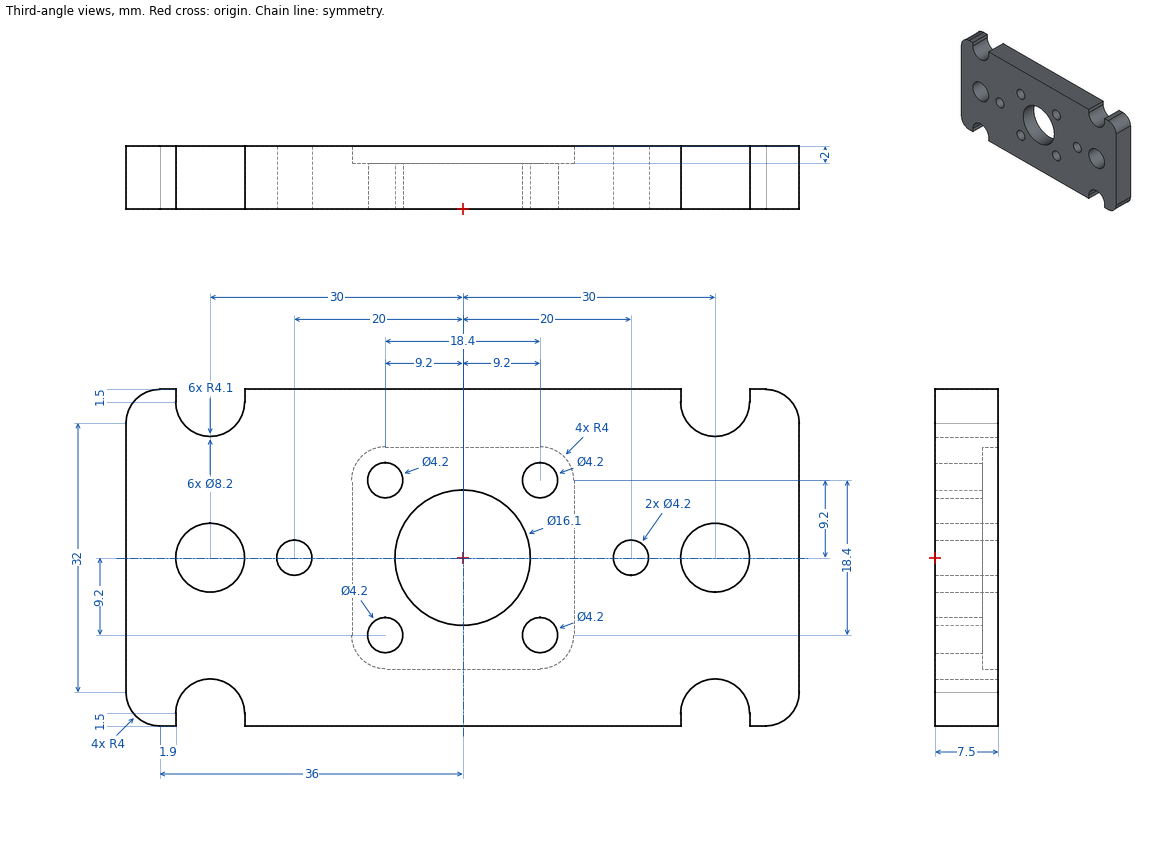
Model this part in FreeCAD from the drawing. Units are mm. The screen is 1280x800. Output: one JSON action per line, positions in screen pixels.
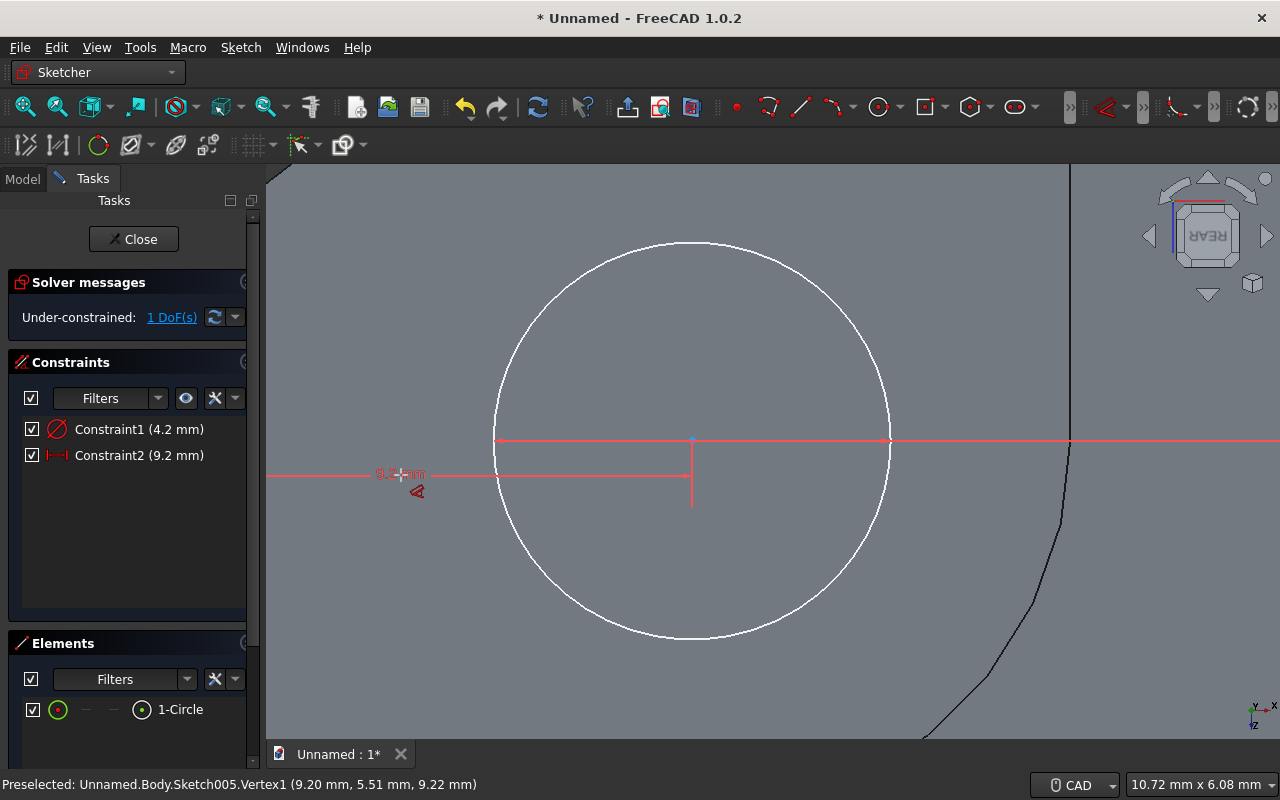
{"action": "left_click", "coordinate": [692, 441]}
{"action": "left_click", "coordinate": [726, 316]}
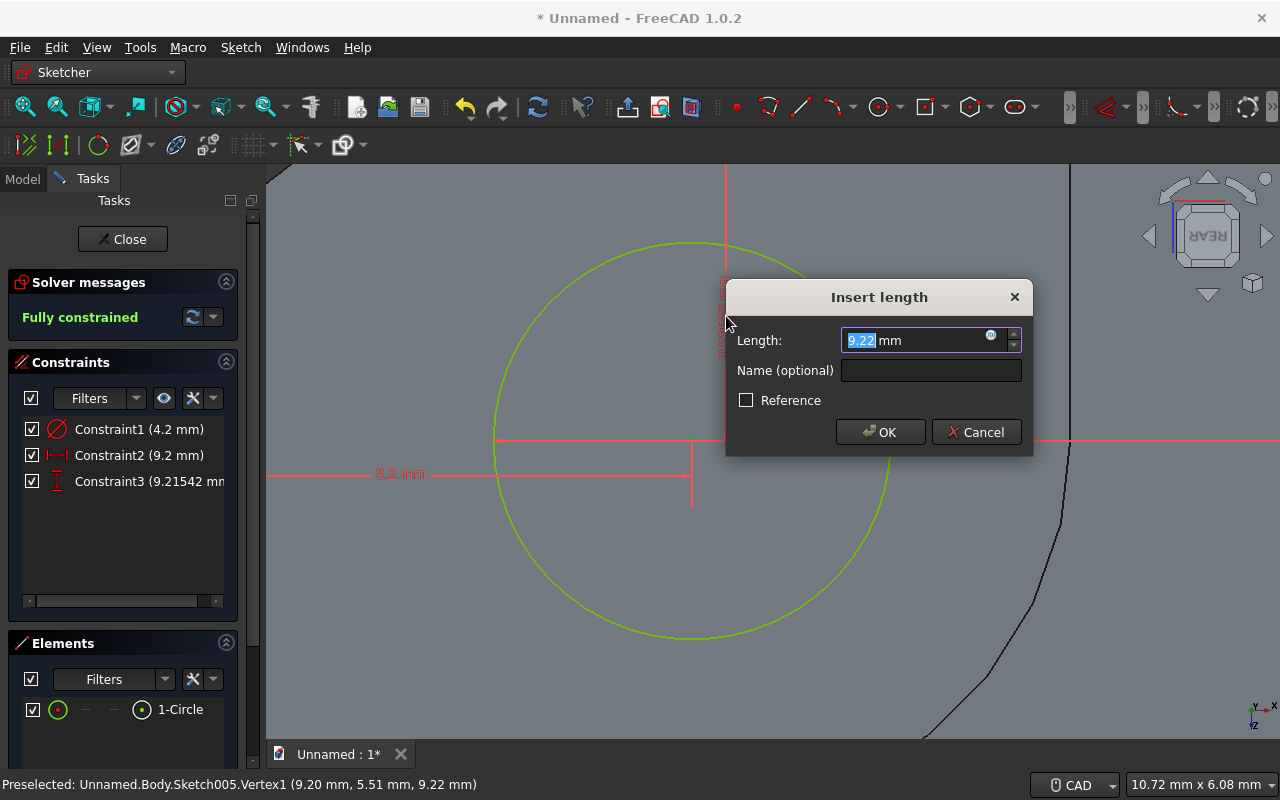
{"action": "type", "text": "9.2"}
{"action": "key", "text": "Return"}
{"action": "key", "text": "Escape"}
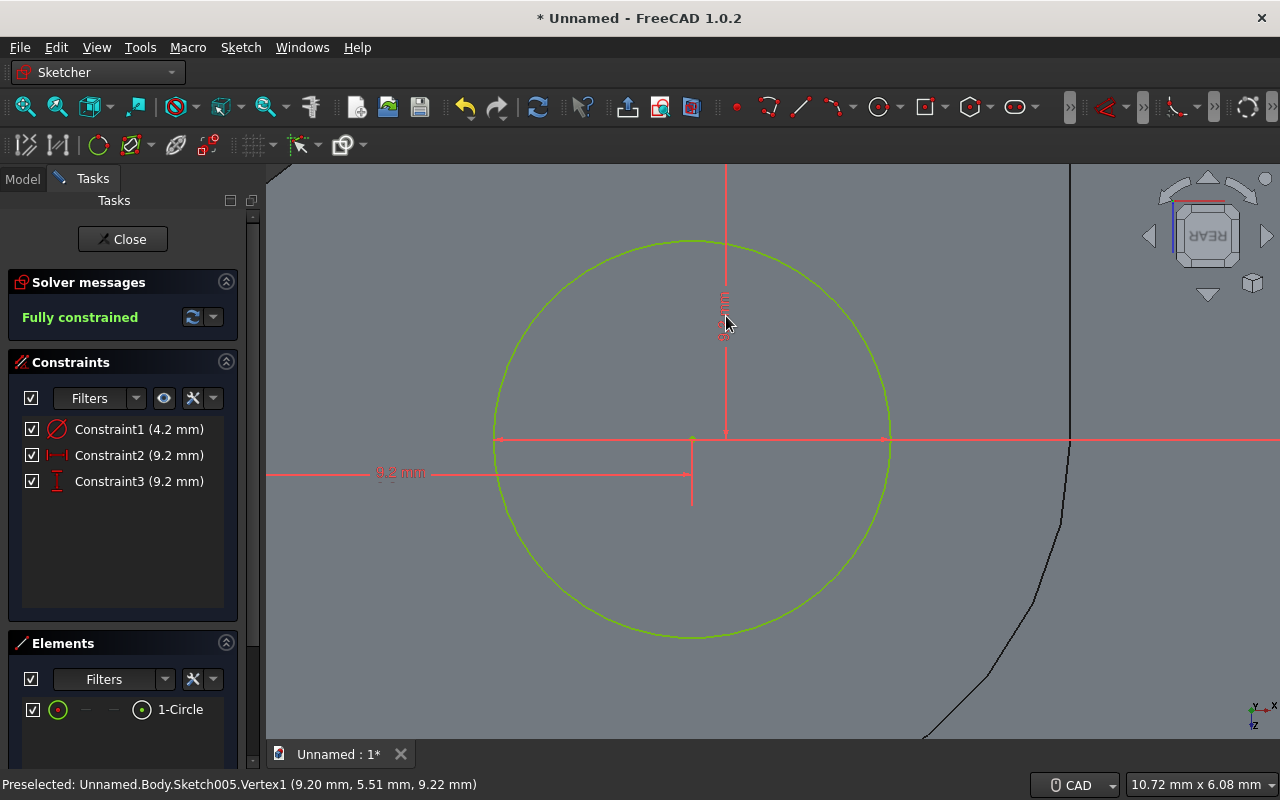
{"action": "left_click", "coordinate": [123, 239]}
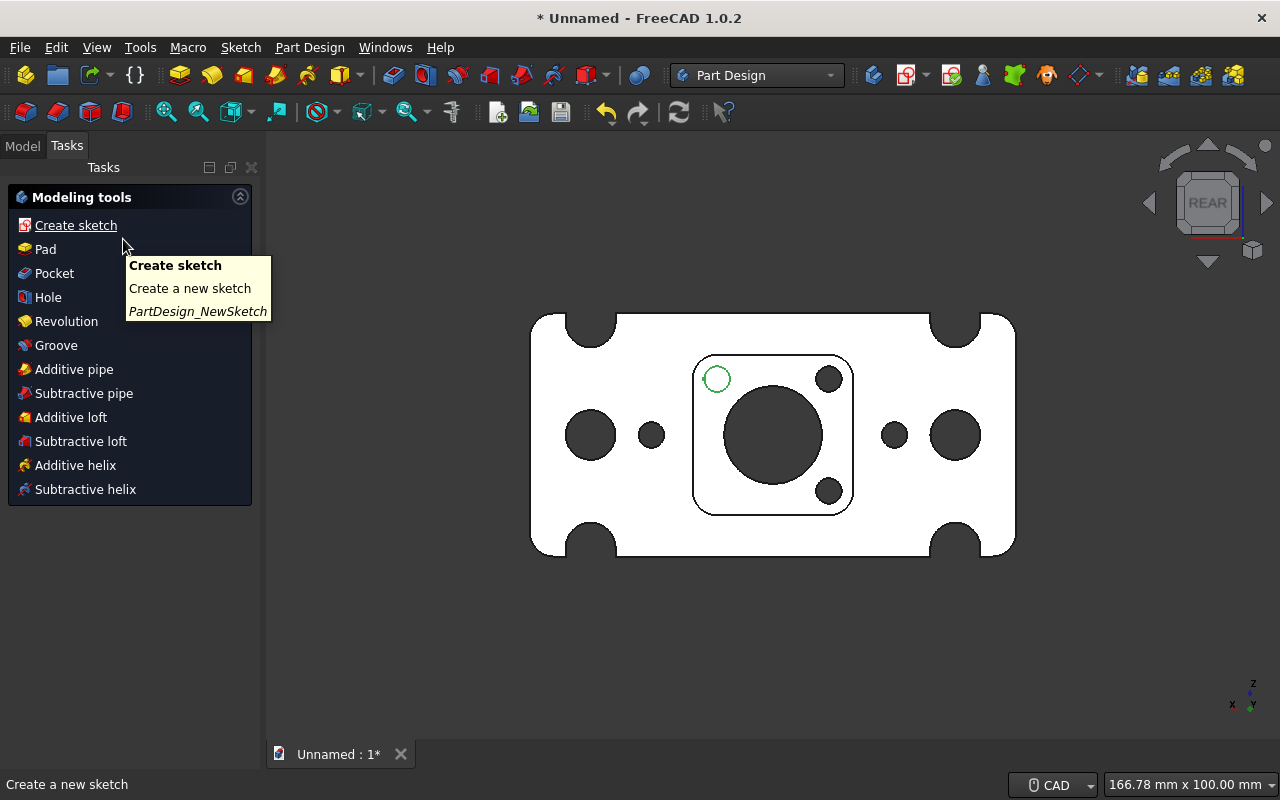
{"action": "left_click", "coordinate": [394, 76]}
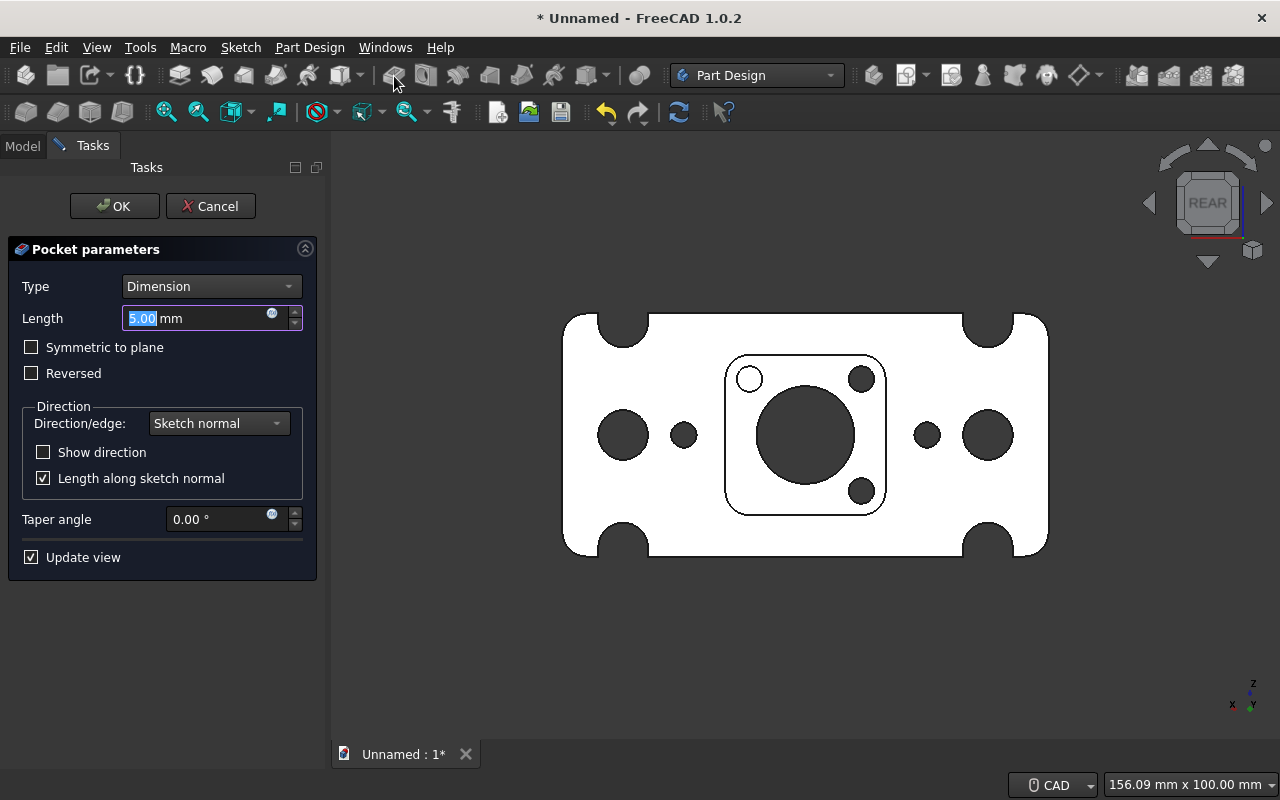
{"action": "left_click", "coordinate": [212, 286]}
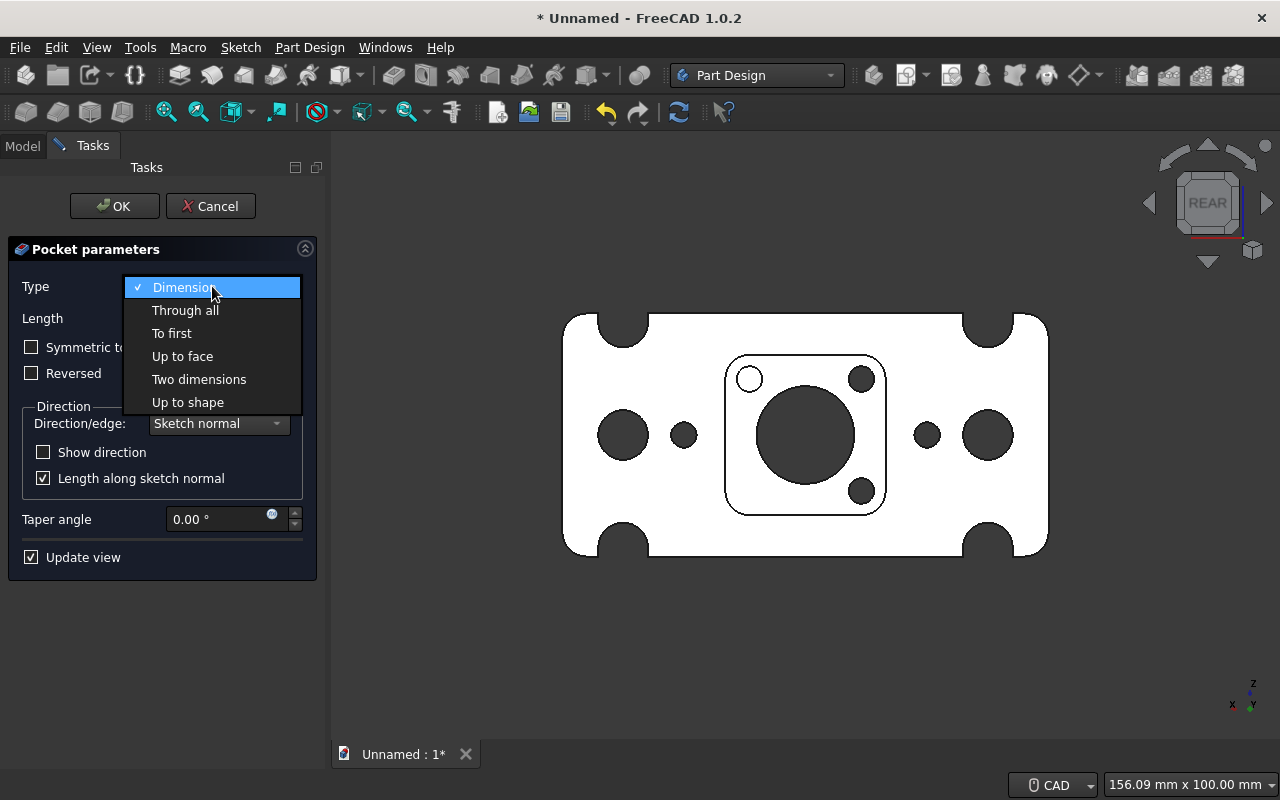
{"action": "left_click", "coordinate": [212, 334]}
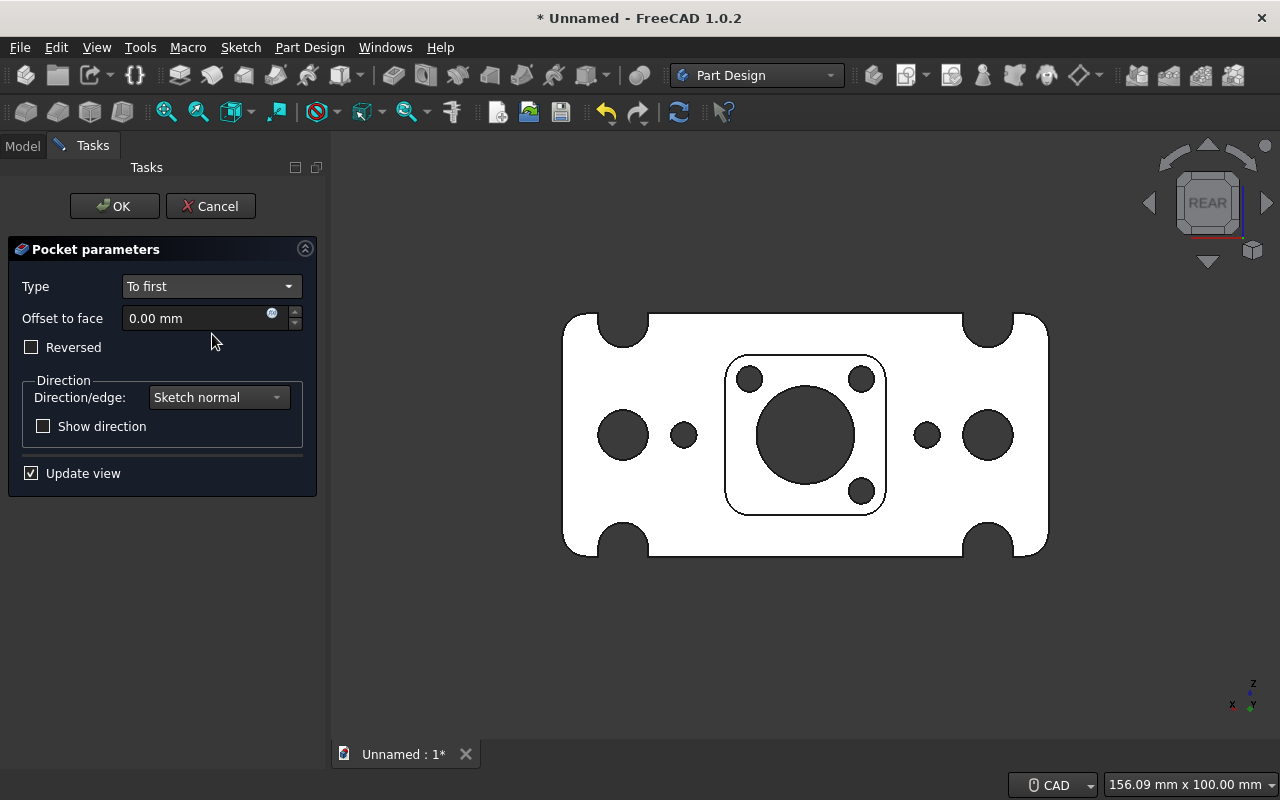
{"action": "left_click", "coordinate": [115, 206]}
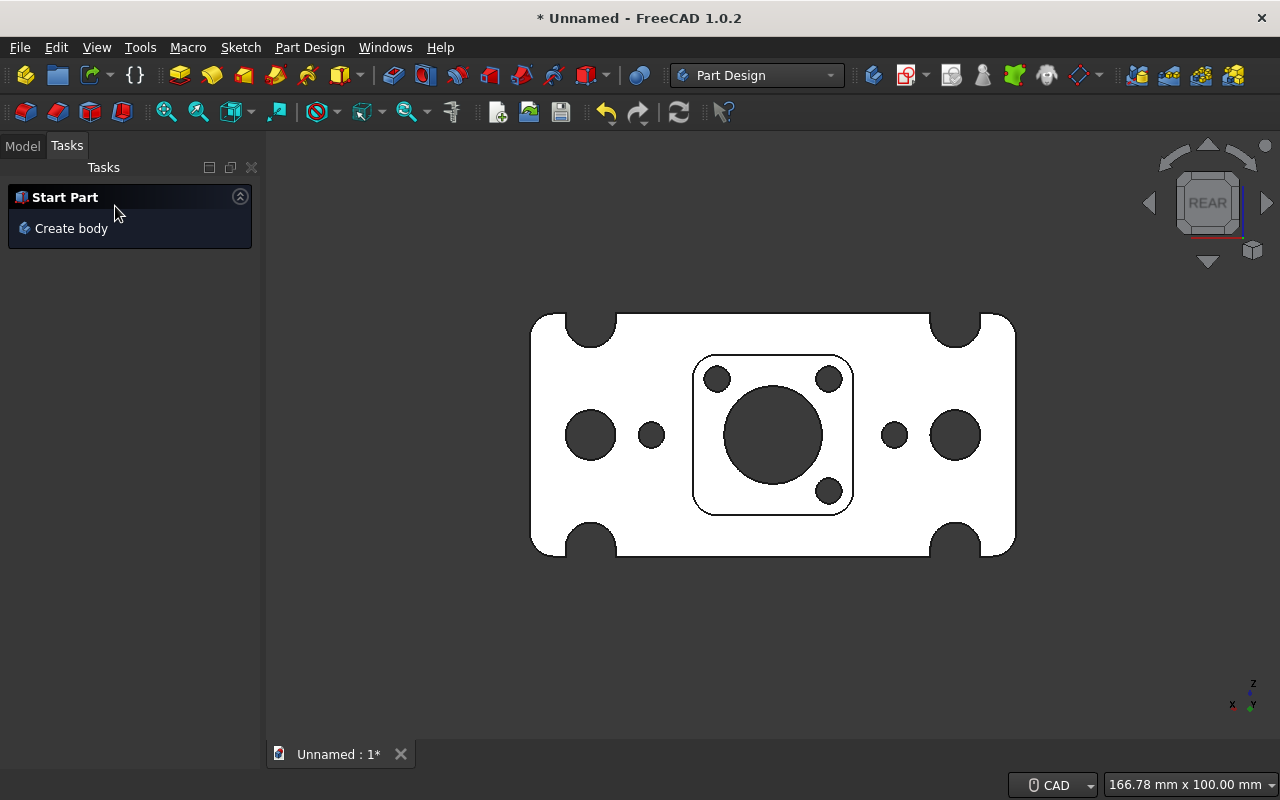
{"action": "left_click", "coordinate": [727, 480]}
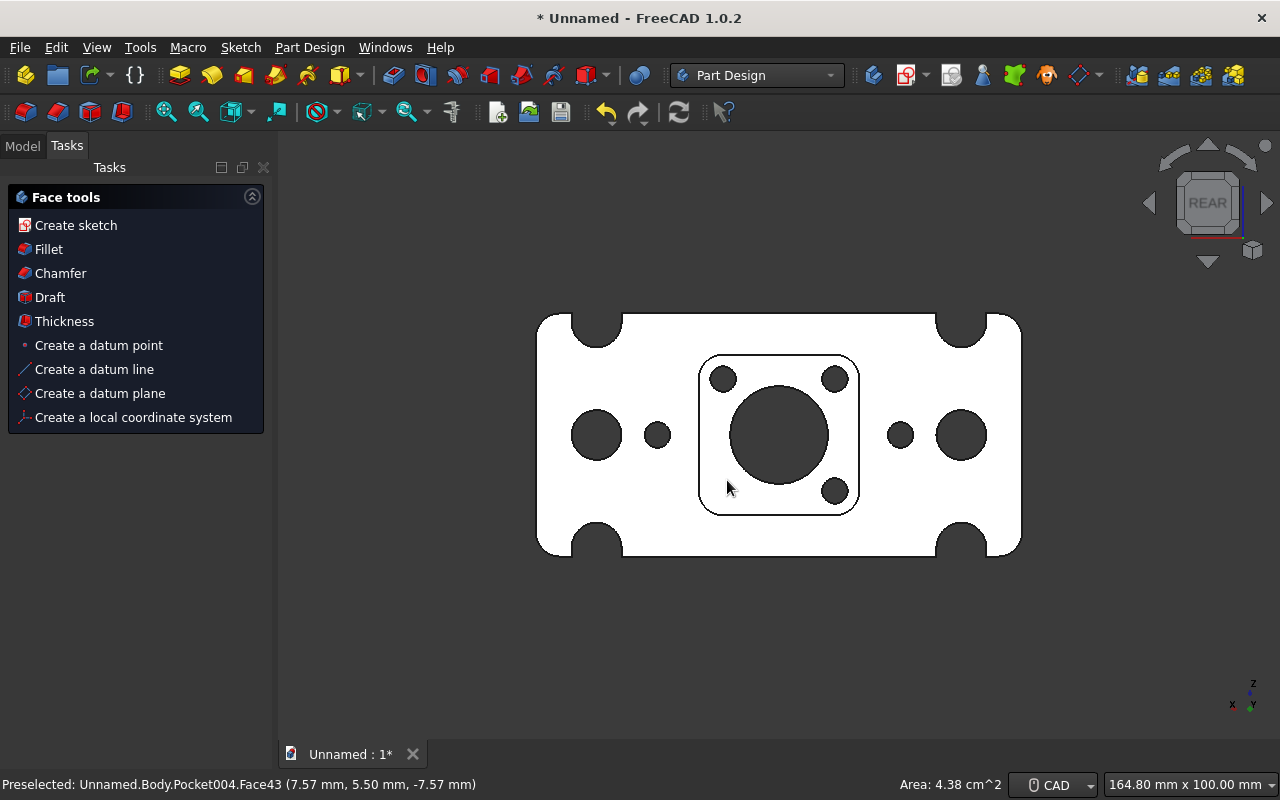
{"action": "left_click", "coordinate": [906, 76]}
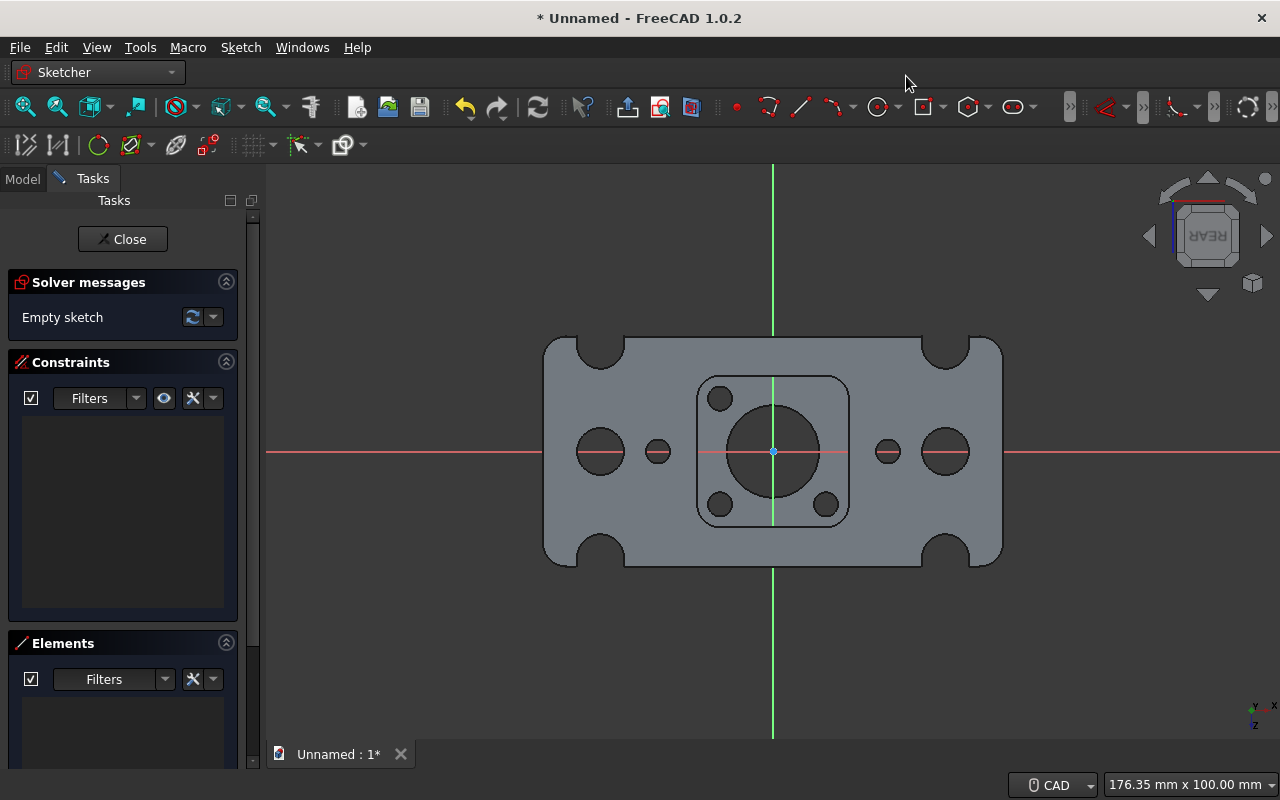
{"action": "scroll", "coordinate": [834, 395], "scroll_direction": "up", "scroll_amount": 14}